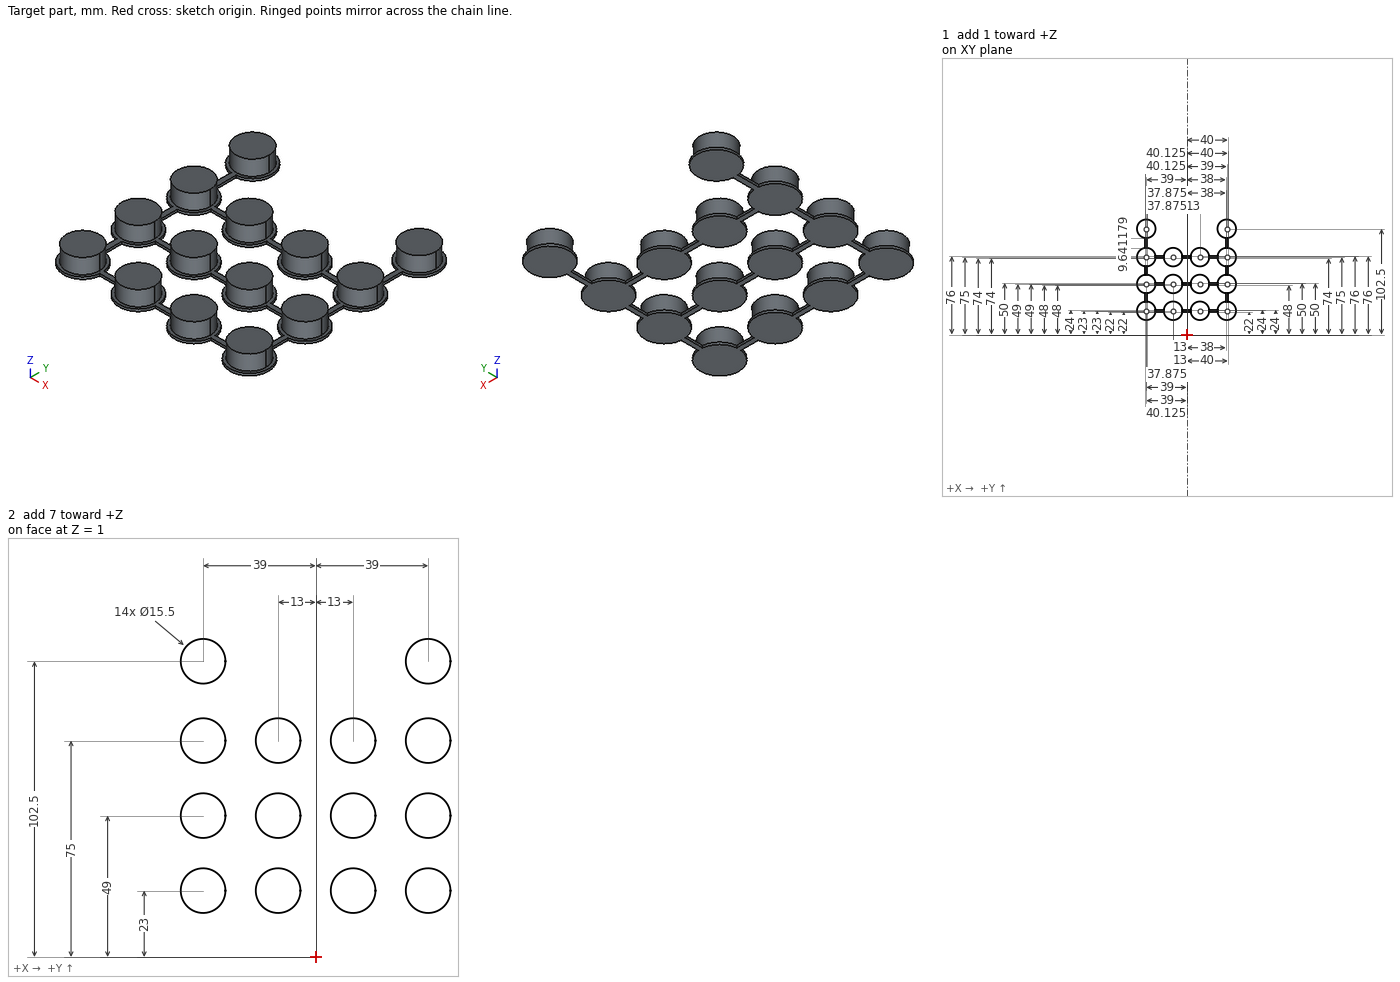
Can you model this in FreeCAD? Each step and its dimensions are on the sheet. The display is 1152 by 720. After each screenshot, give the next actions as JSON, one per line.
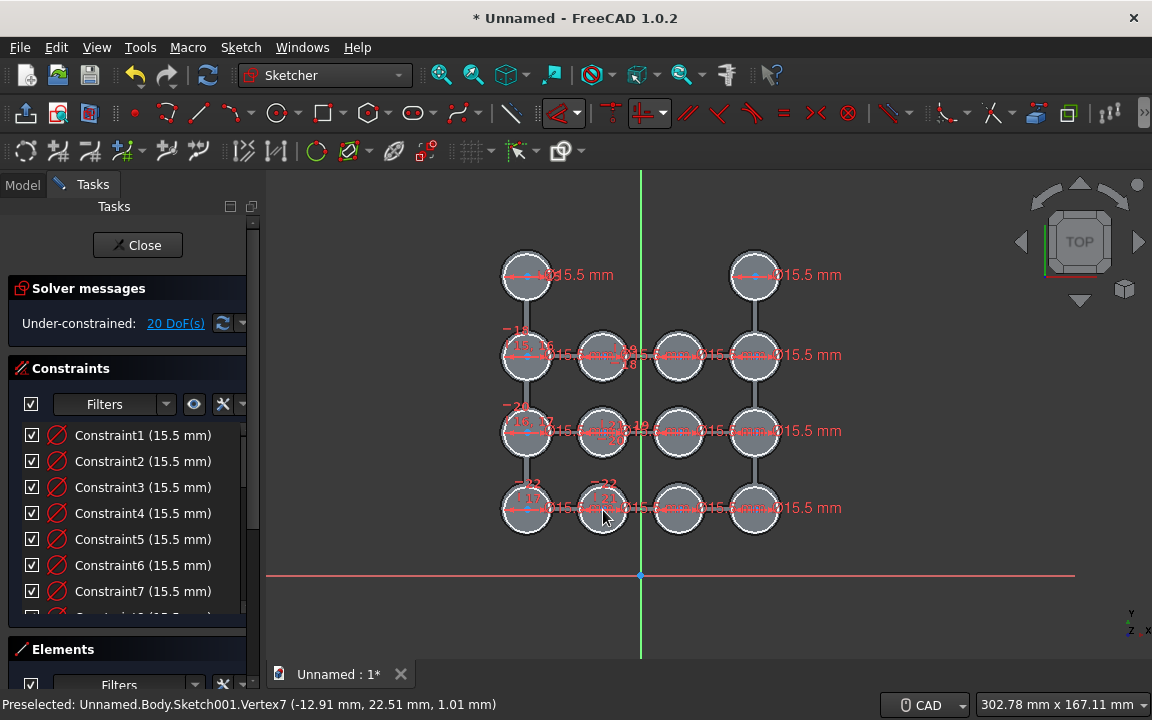
{"action": "left_click", "coordinate": [603, 357]}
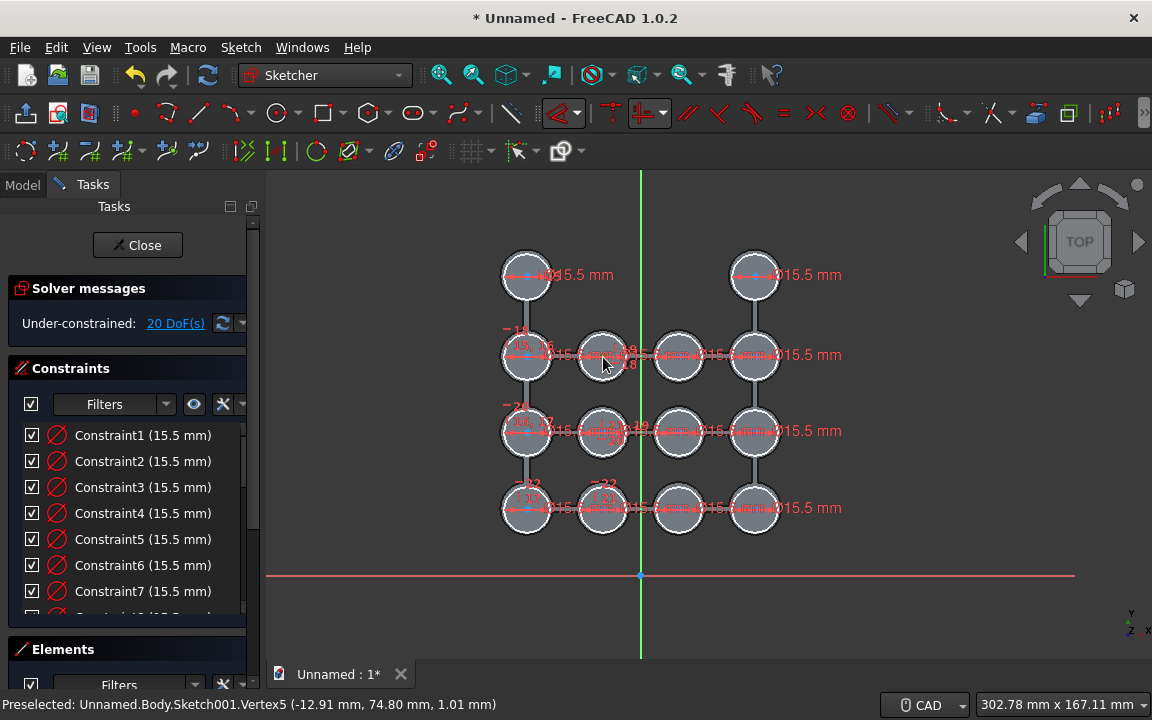
{"action": "left_click", "coordinate": [679, 357]}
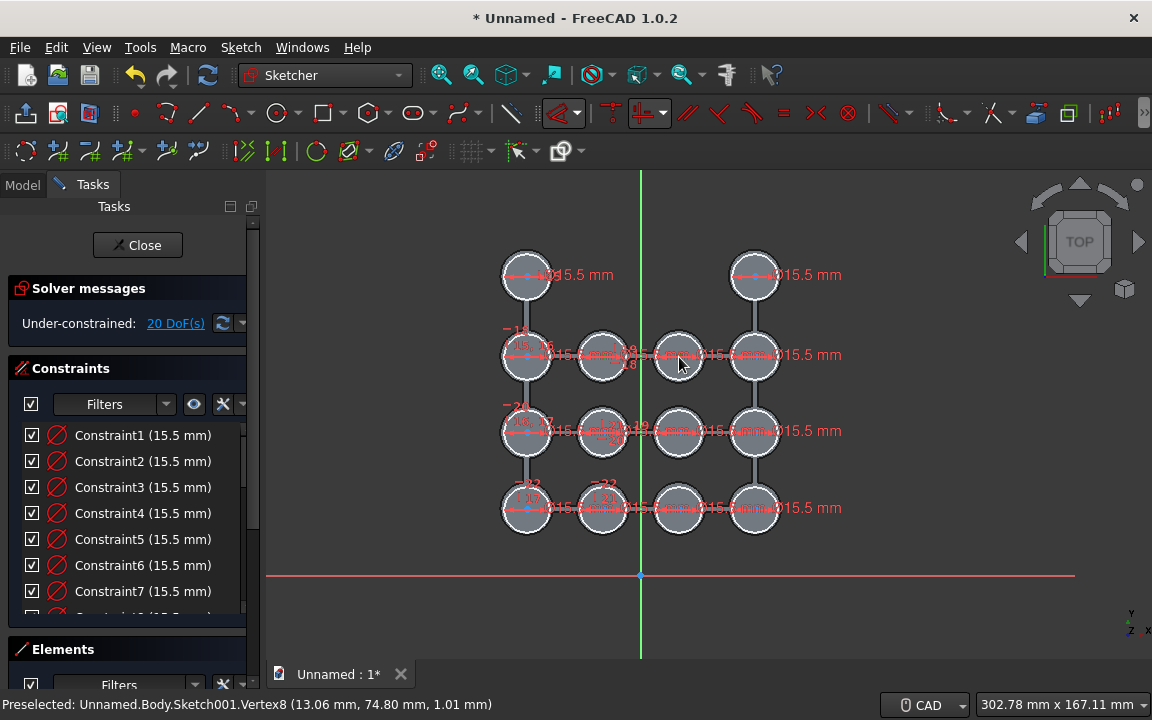
{"action": "left_click", "coordinate": [666, 114]}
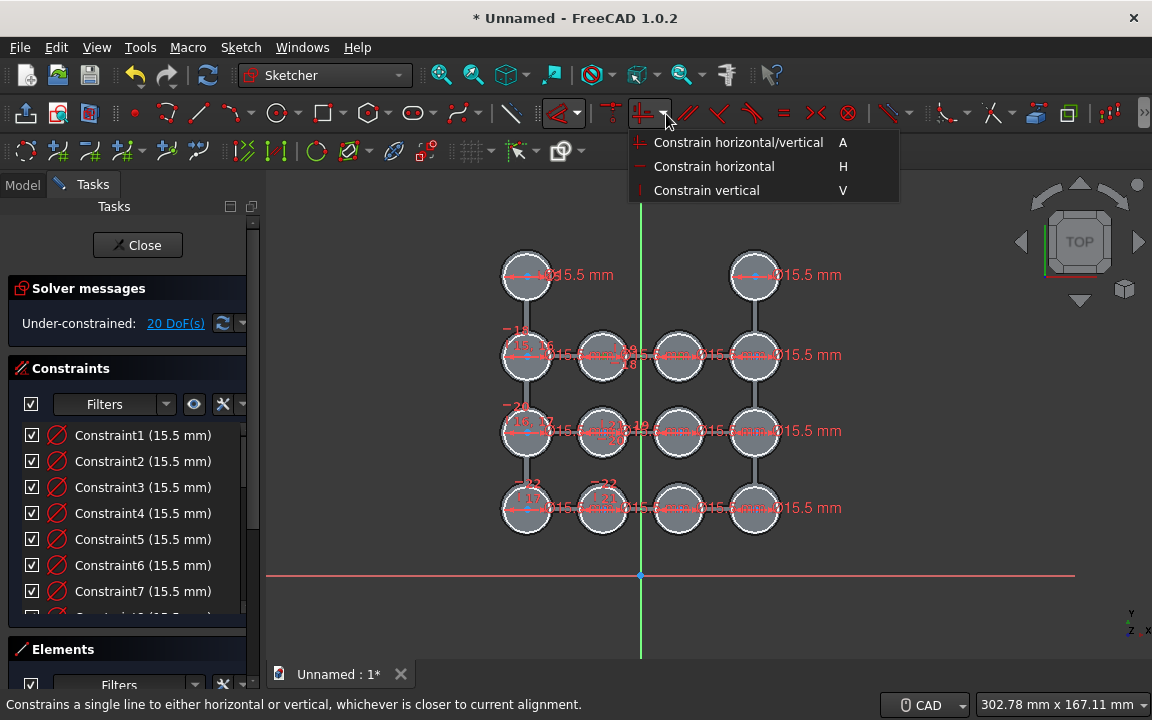
{"action": "left_click", "coordinate": [764, 166]}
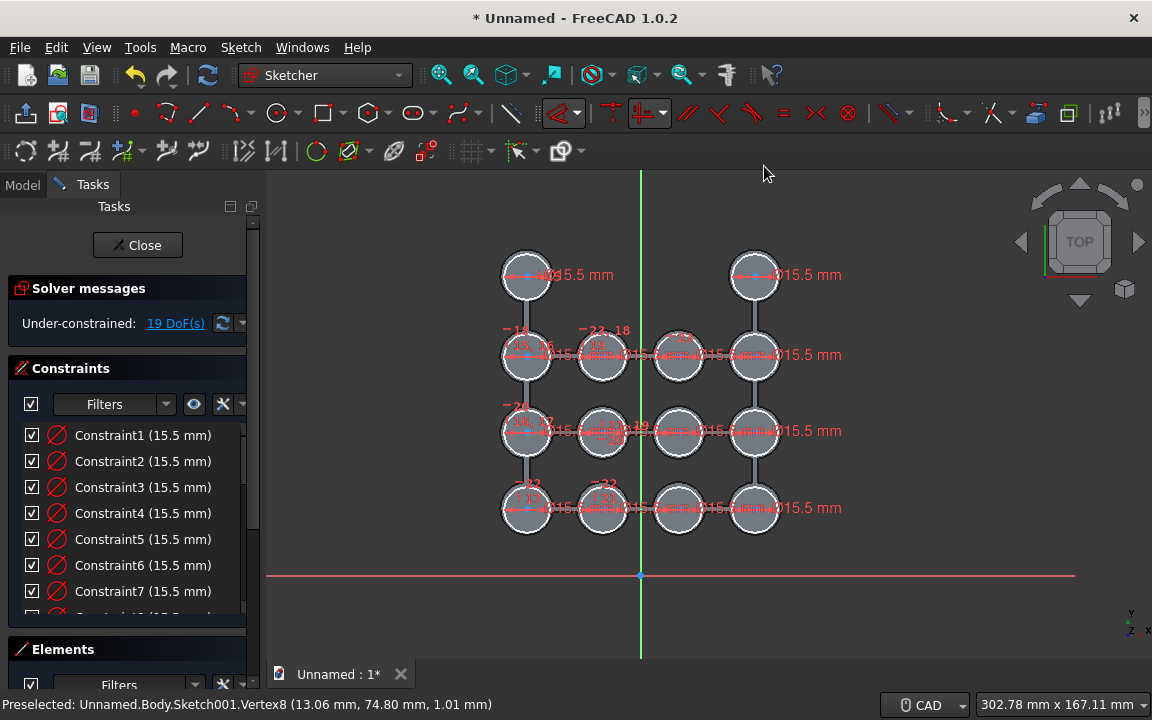
{"action": "left_click", "coordinate": [527, 277]}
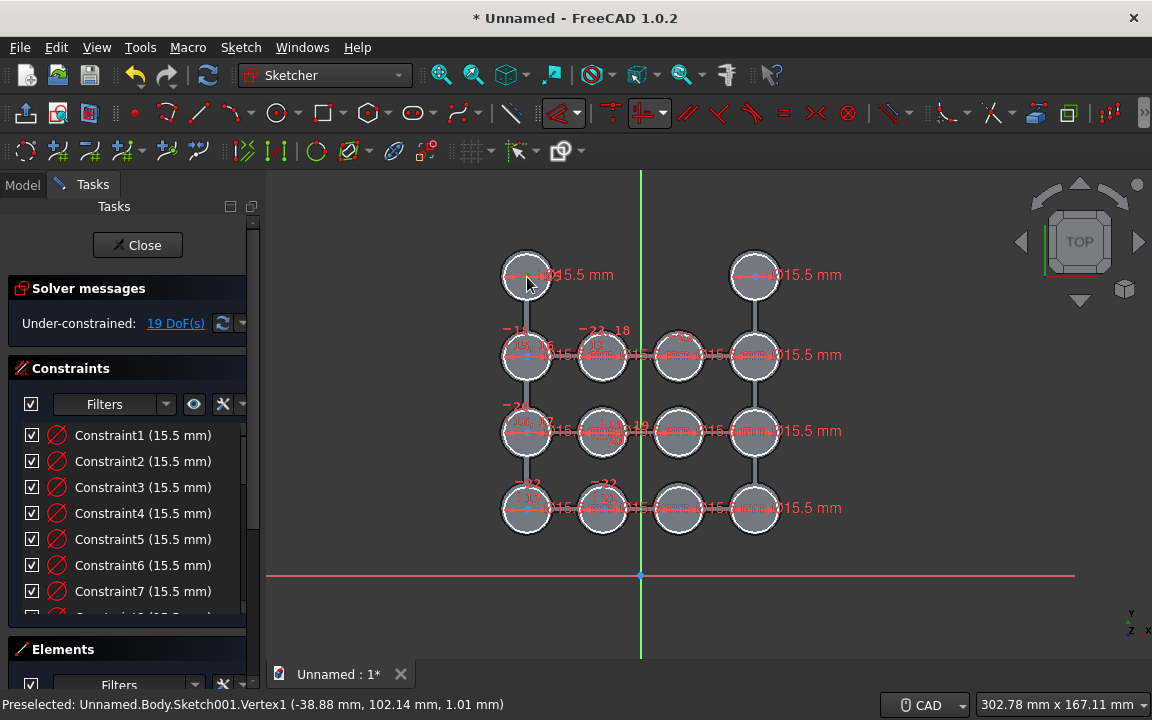
{"action": "left_click", "coordinate": [755, 277]}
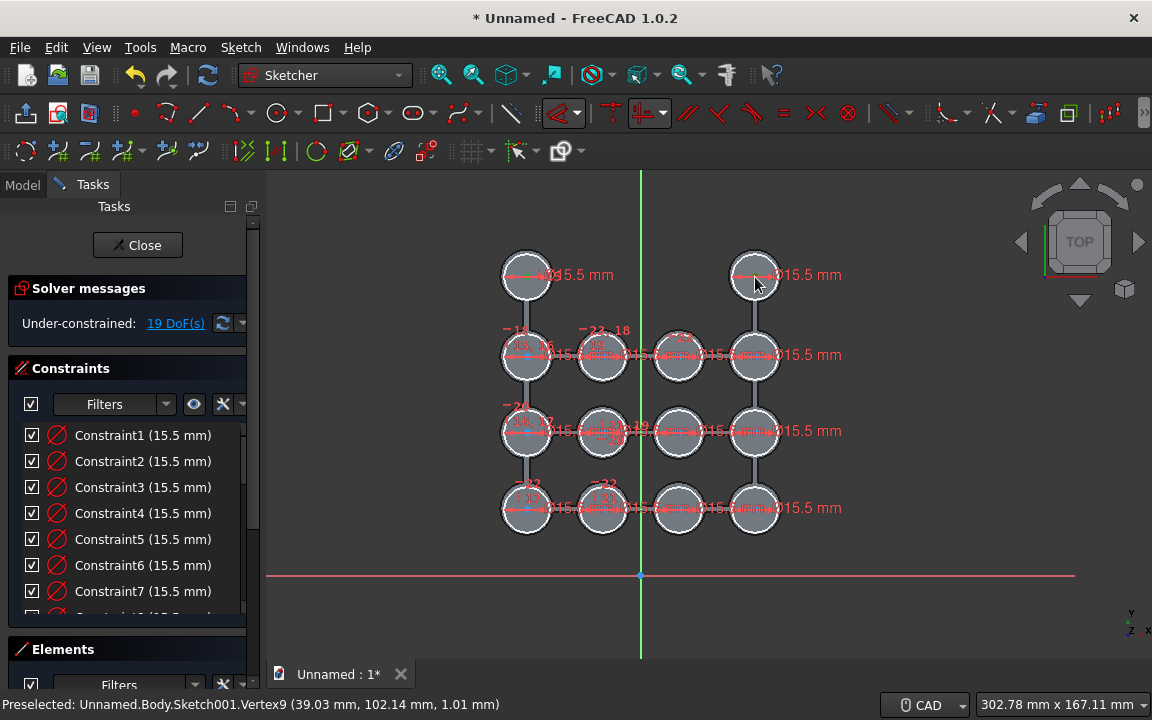
{"action": "key", "text": "h"}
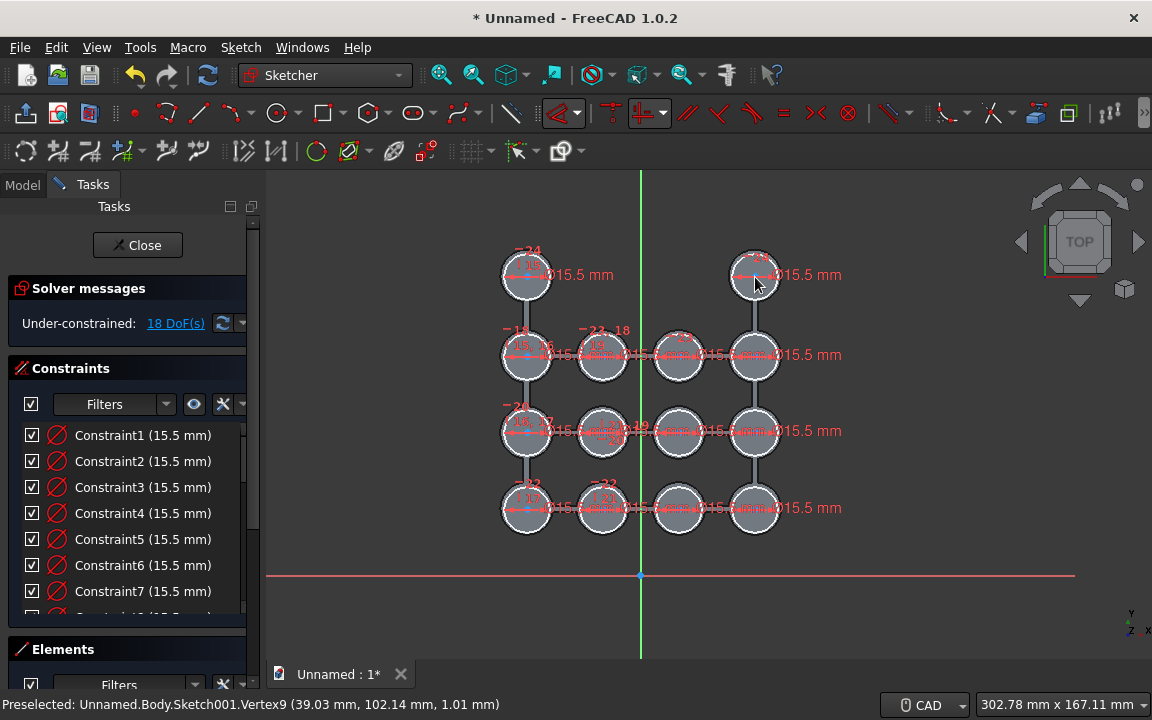
{"action": "left_click", "coordinate": [755, 277]}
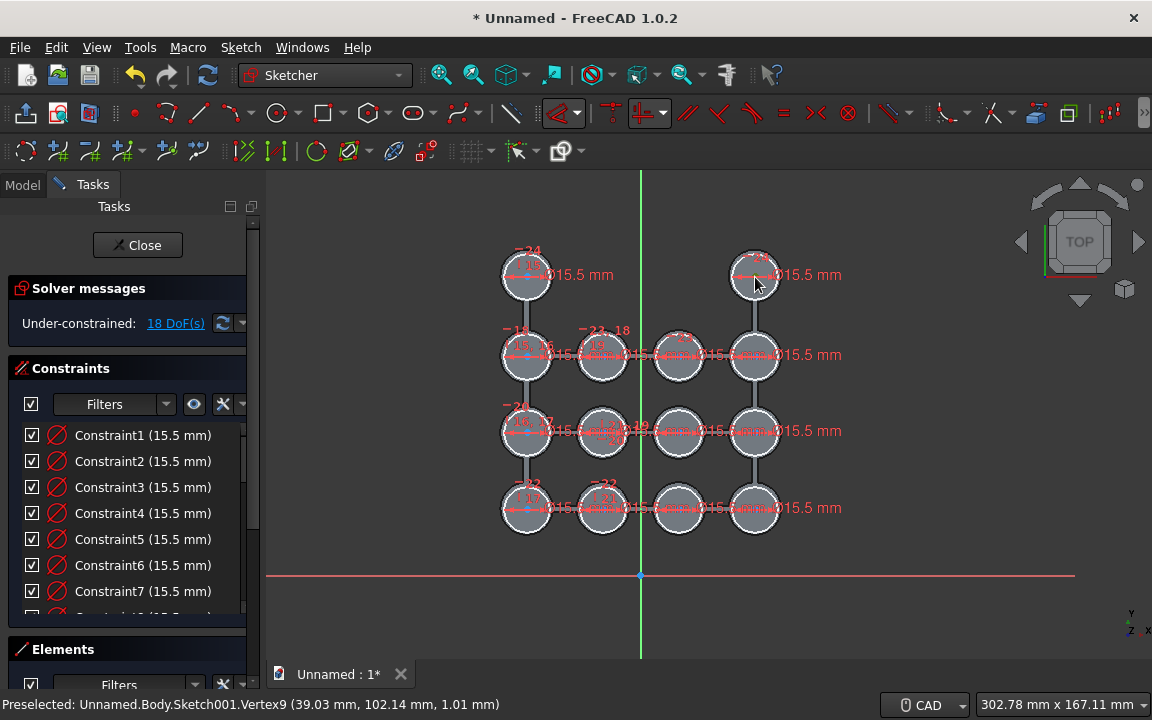
{"action": "left_click", "coordinate": [755, 510]}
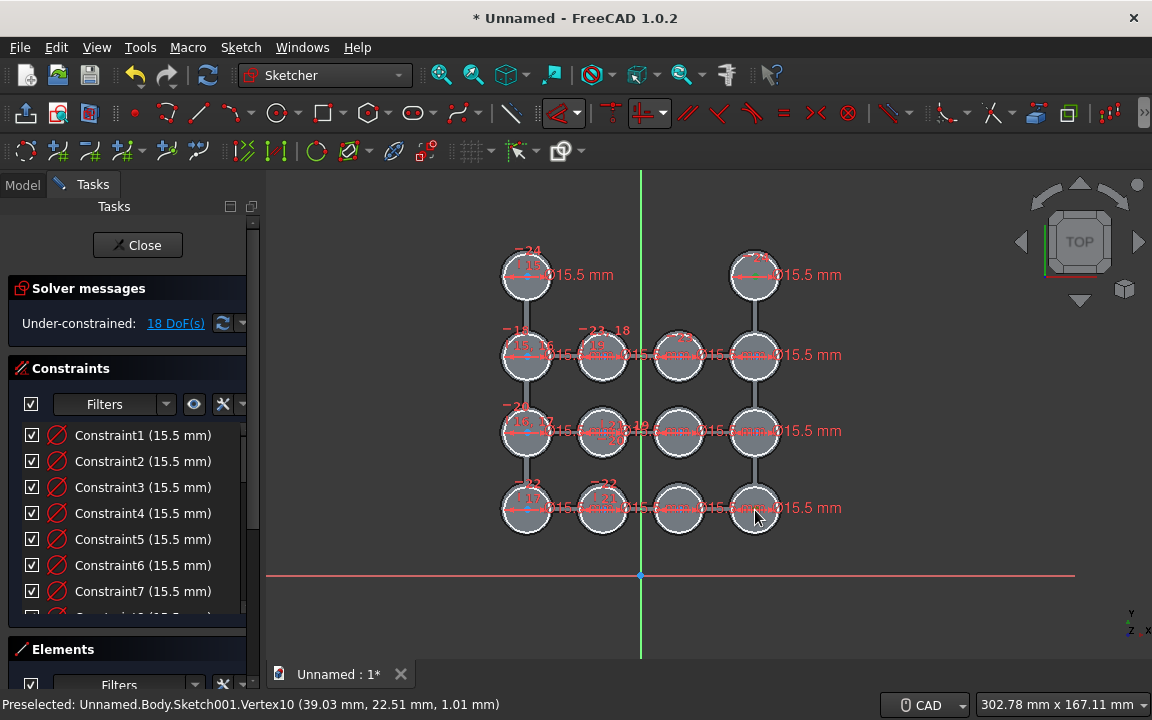
{"action": "left_click", "coordinate": [666, 114]}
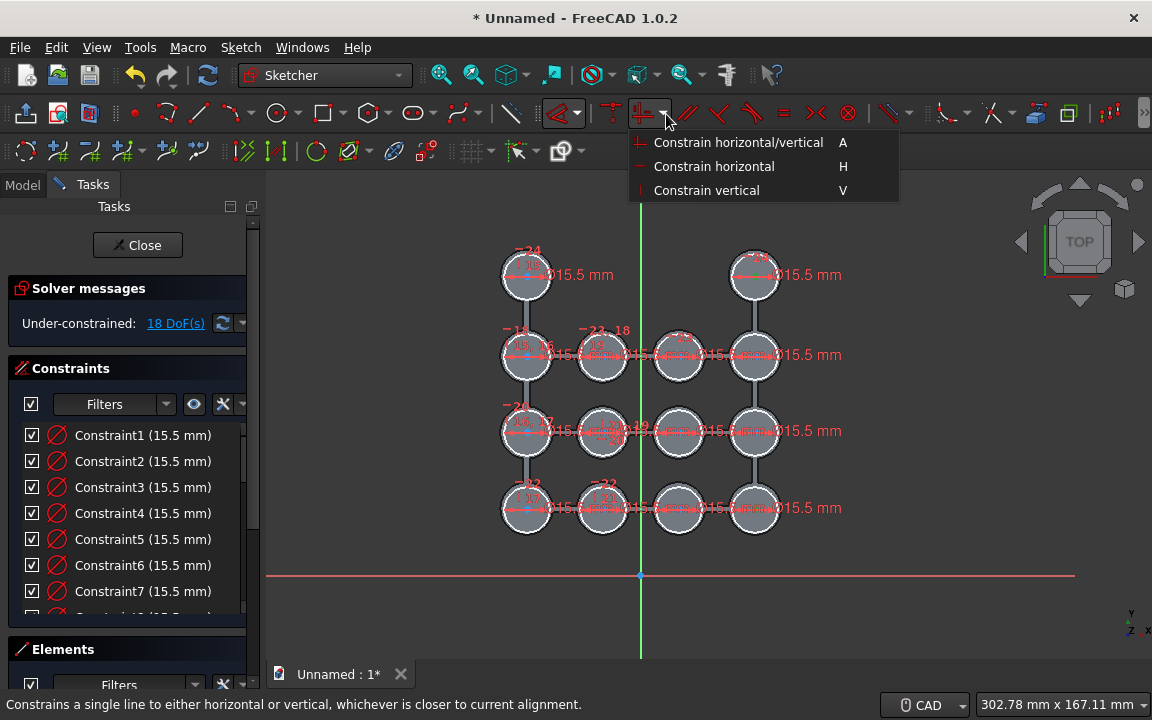
{"action": "left_click", "coordinate": [764, 190]}